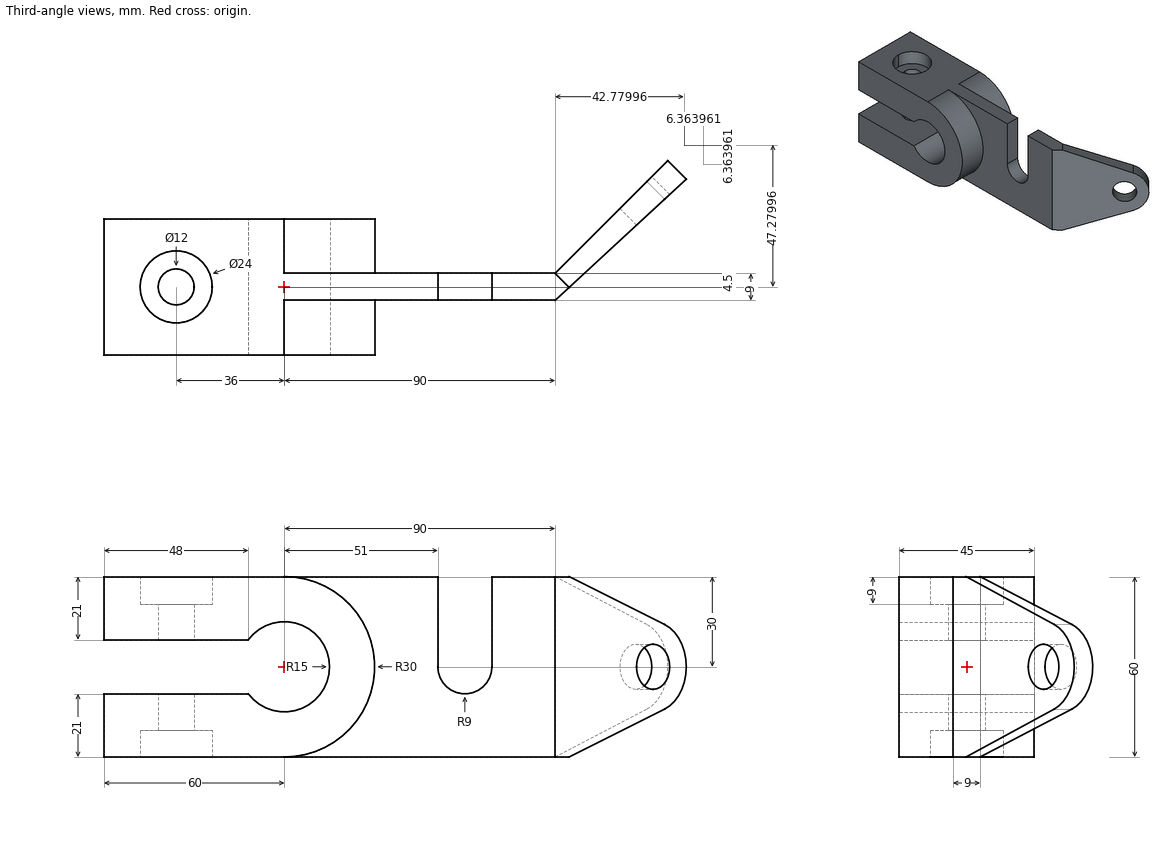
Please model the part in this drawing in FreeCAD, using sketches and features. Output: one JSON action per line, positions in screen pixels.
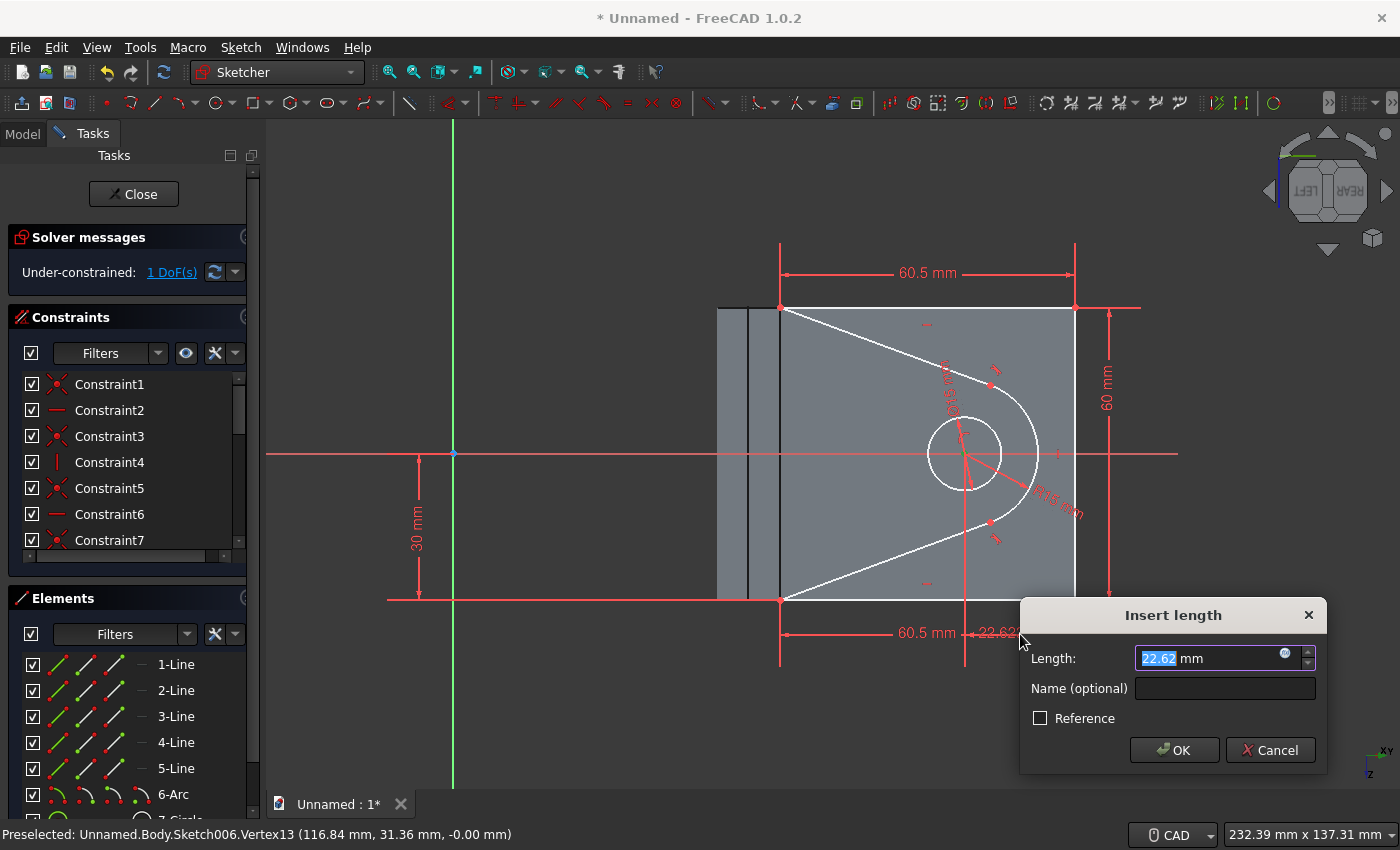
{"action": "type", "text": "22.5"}
{"action": "key", "text": "Return"}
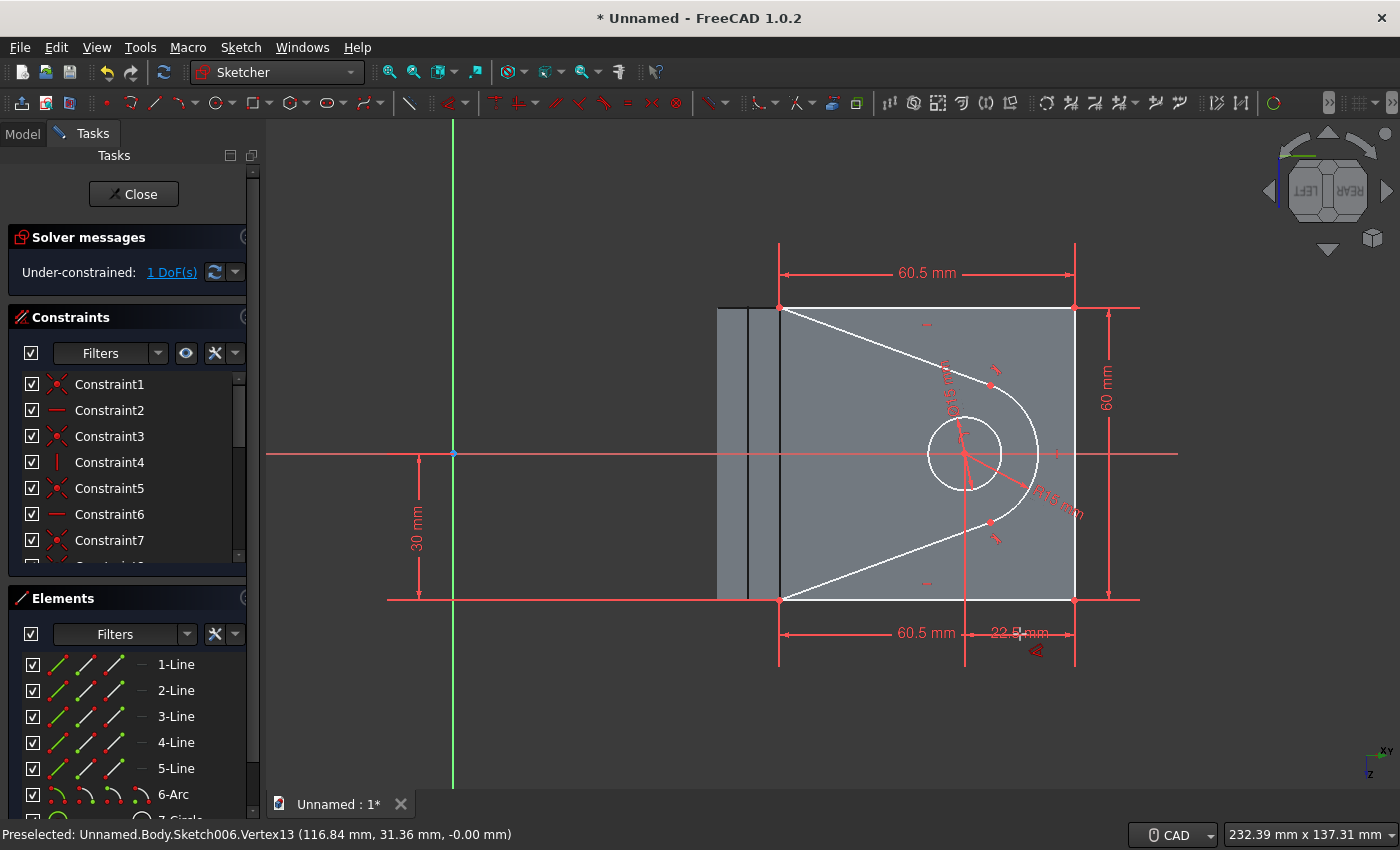
{"action": "left_click", "coordinate": [779, 600]}
{"action": "left_click", "coordinate": [616, 634]}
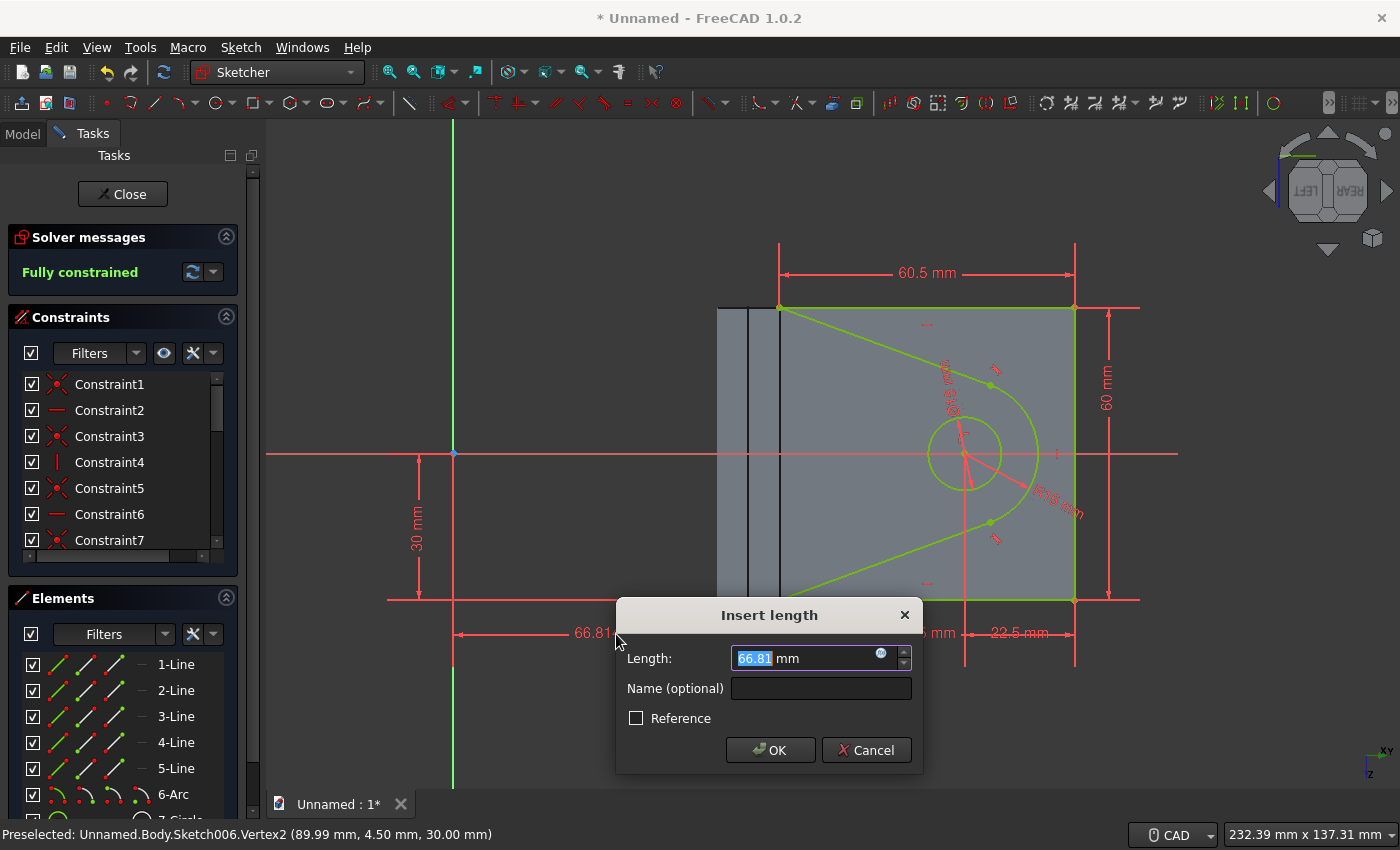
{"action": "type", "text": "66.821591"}
{"action": "key", "text": "Return"}
{"action": "key", "text": "Escape"}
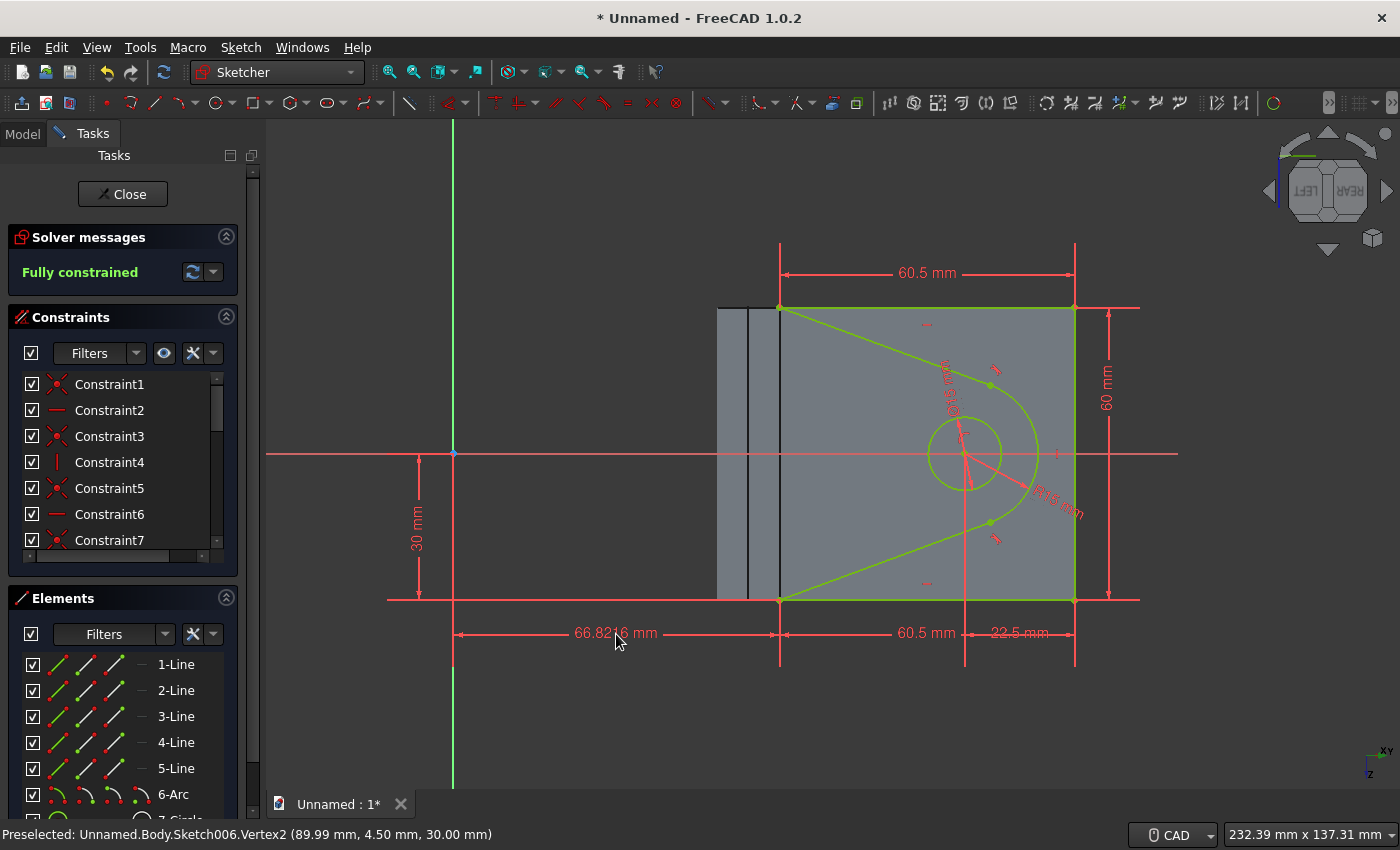
{"action": "left_click", "coordinate": [123, 194]}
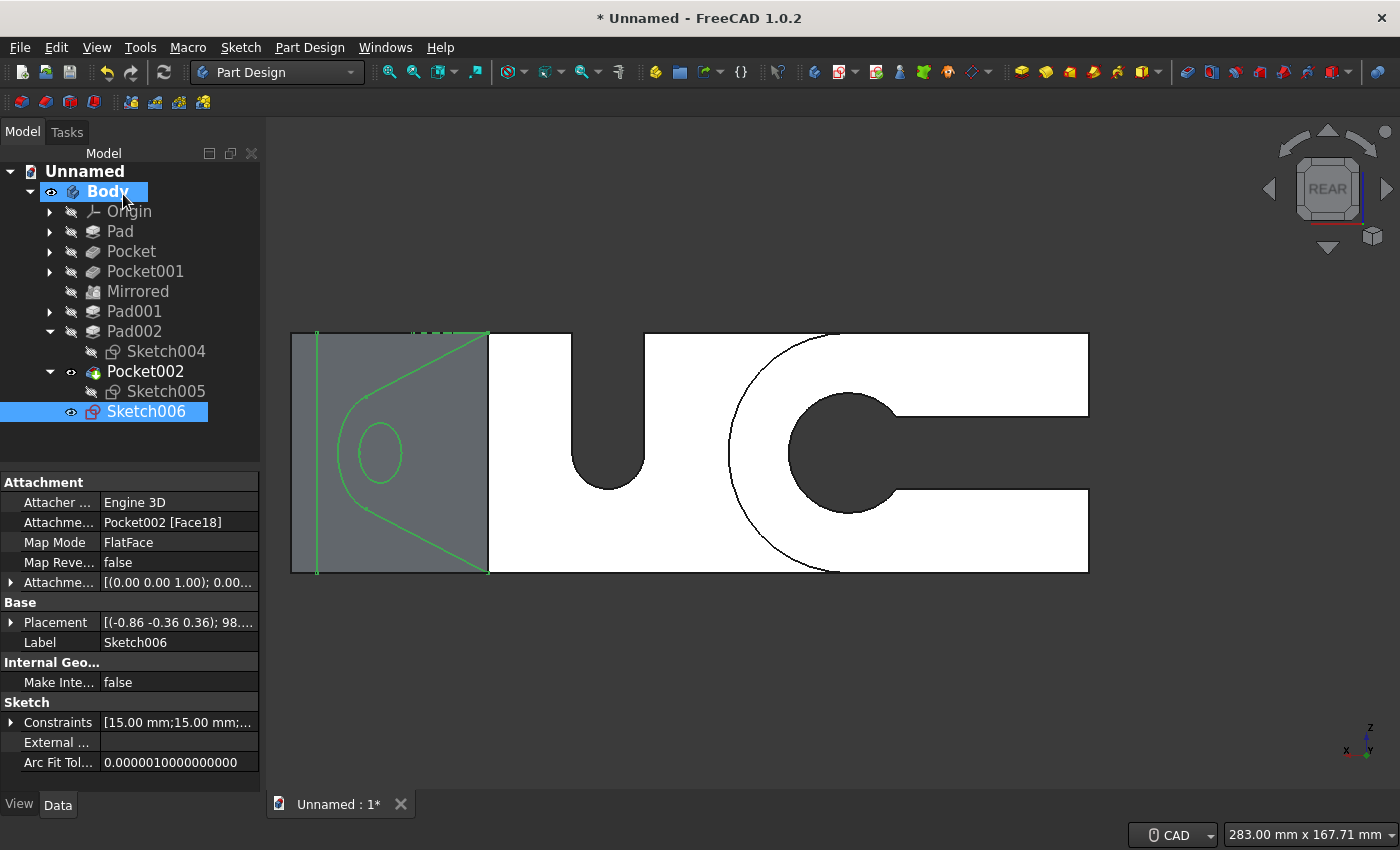
{"action": "left_click", "coordinate": [1188, 72]}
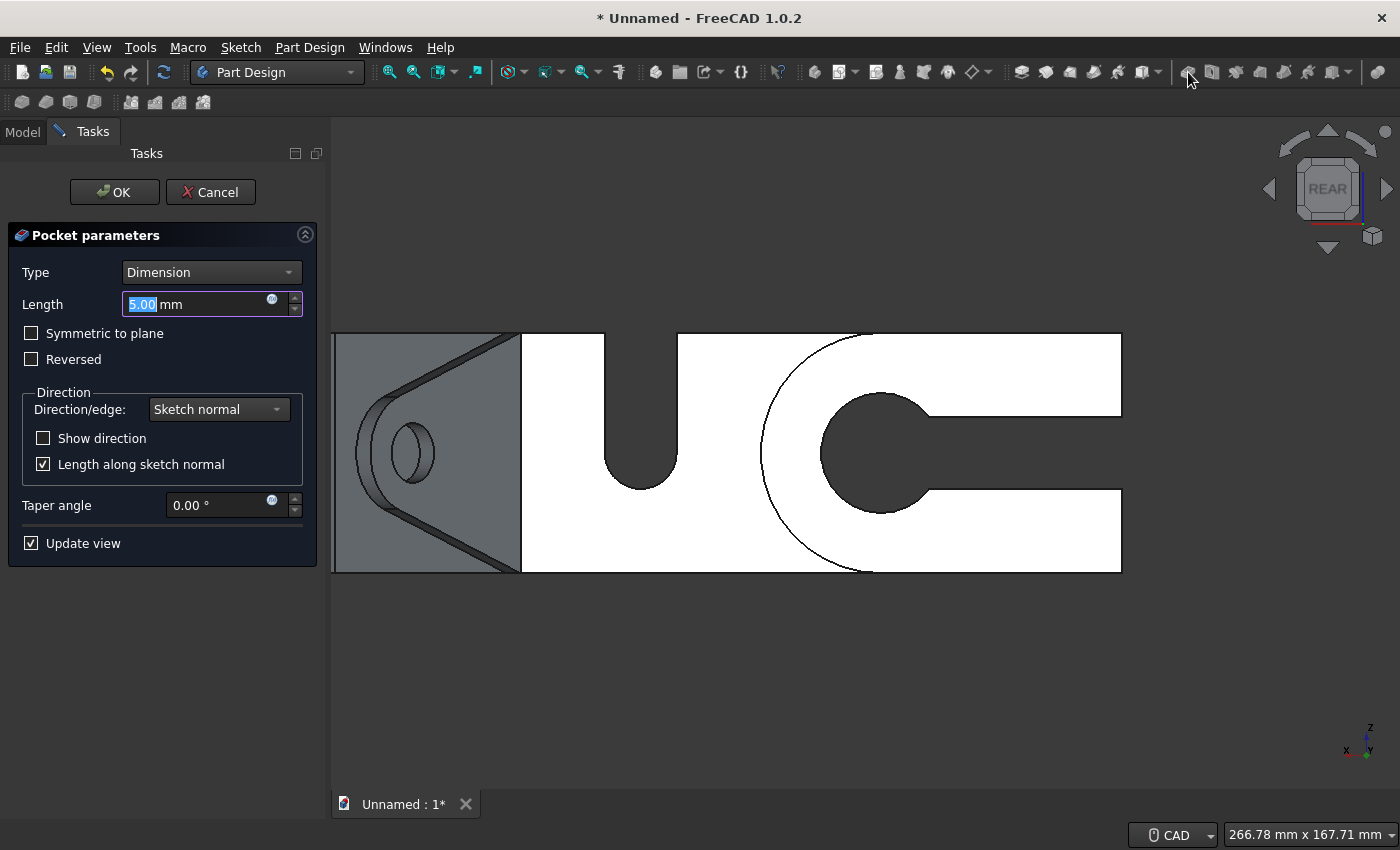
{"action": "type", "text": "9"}
{"action": "key", "text": "Tab"}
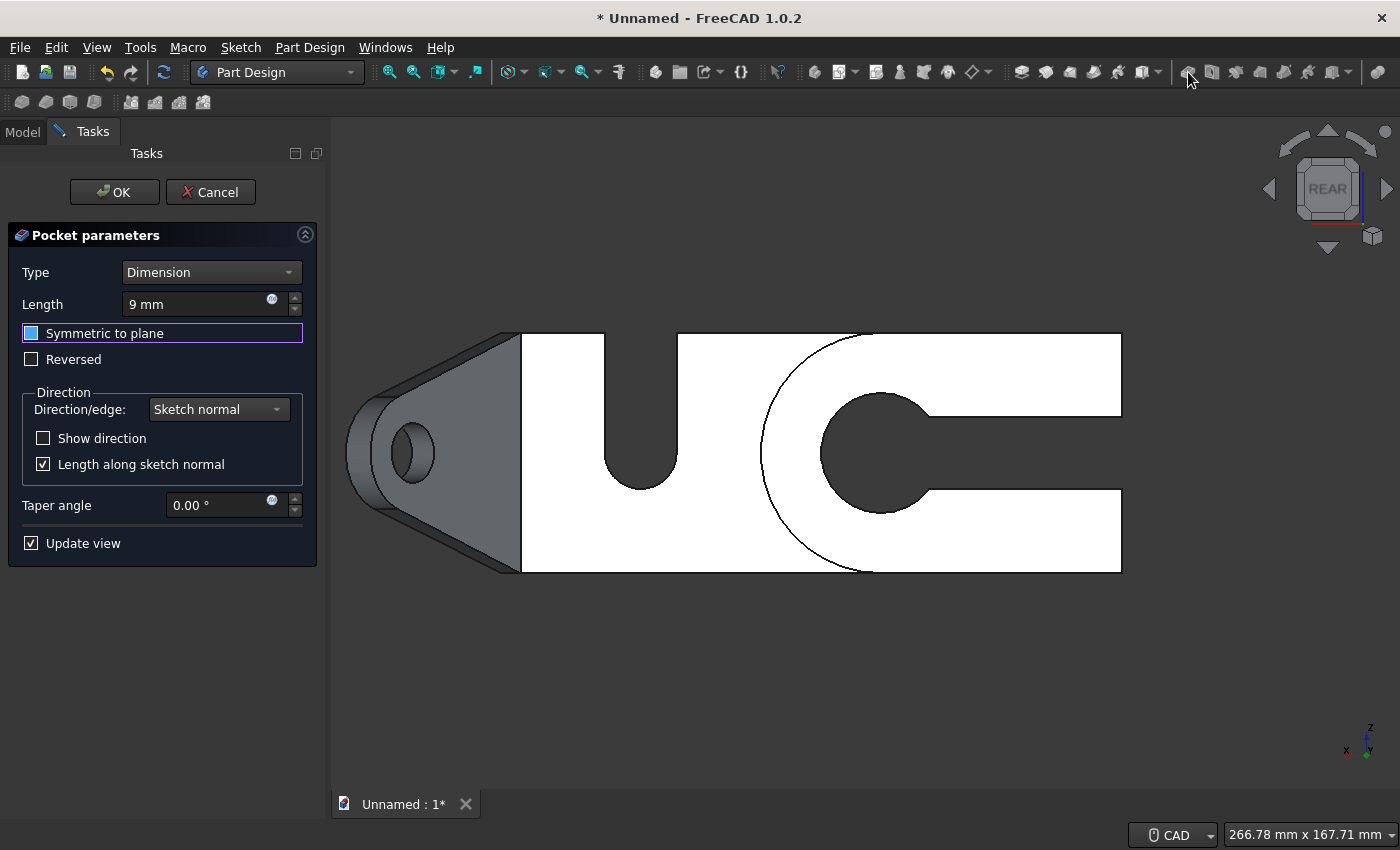
{"action": "left_click", "coordinate": [115, 192]}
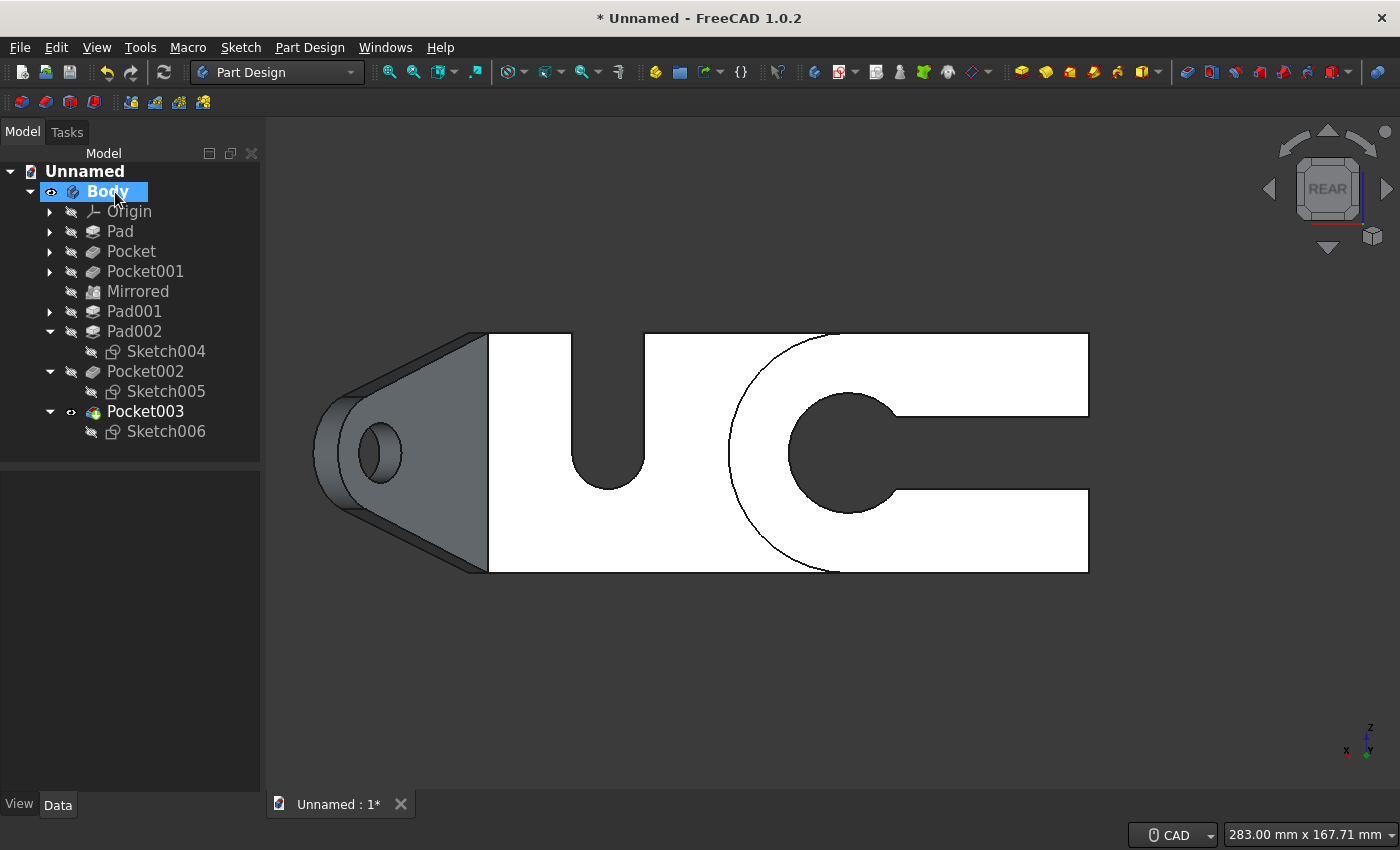
{"action": "key", "text": "0"}